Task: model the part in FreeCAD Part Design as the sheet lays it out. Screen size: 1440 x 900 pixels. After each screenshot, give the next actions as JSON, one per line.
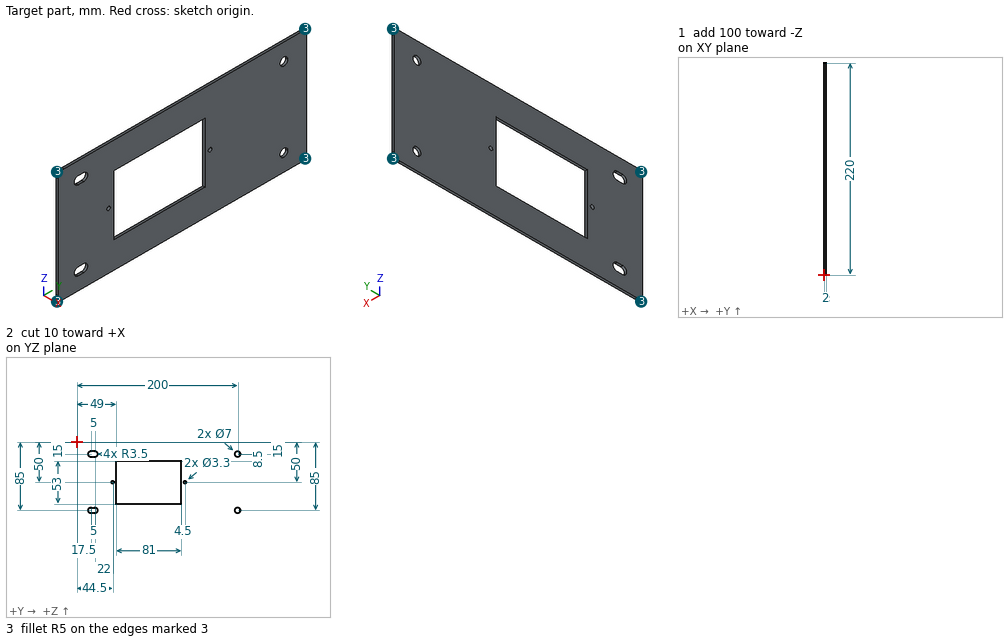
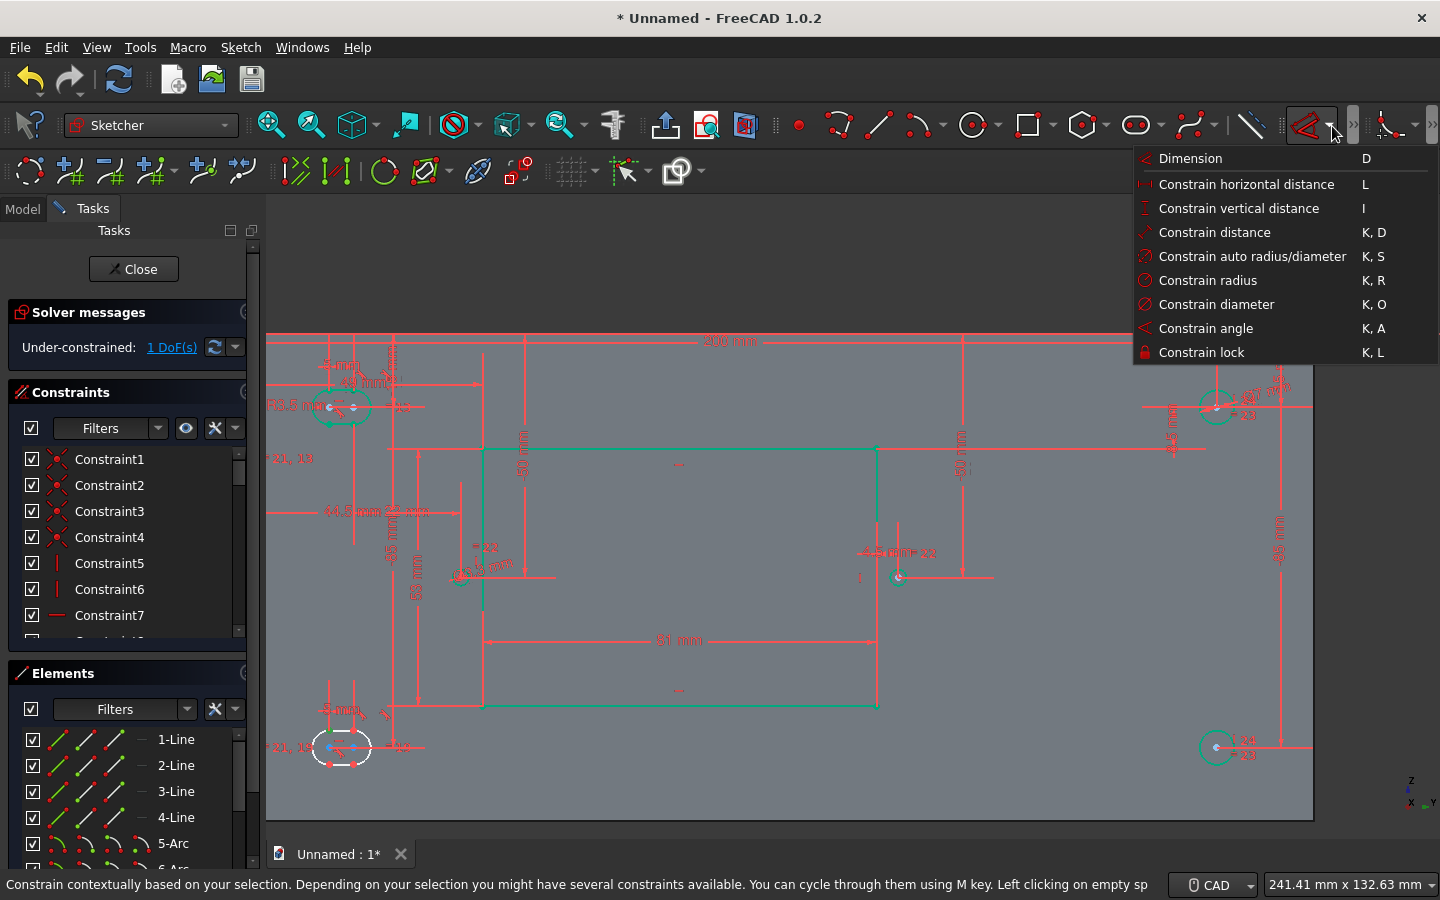
{"action": "left_click", "coordinate": [1286, 184]}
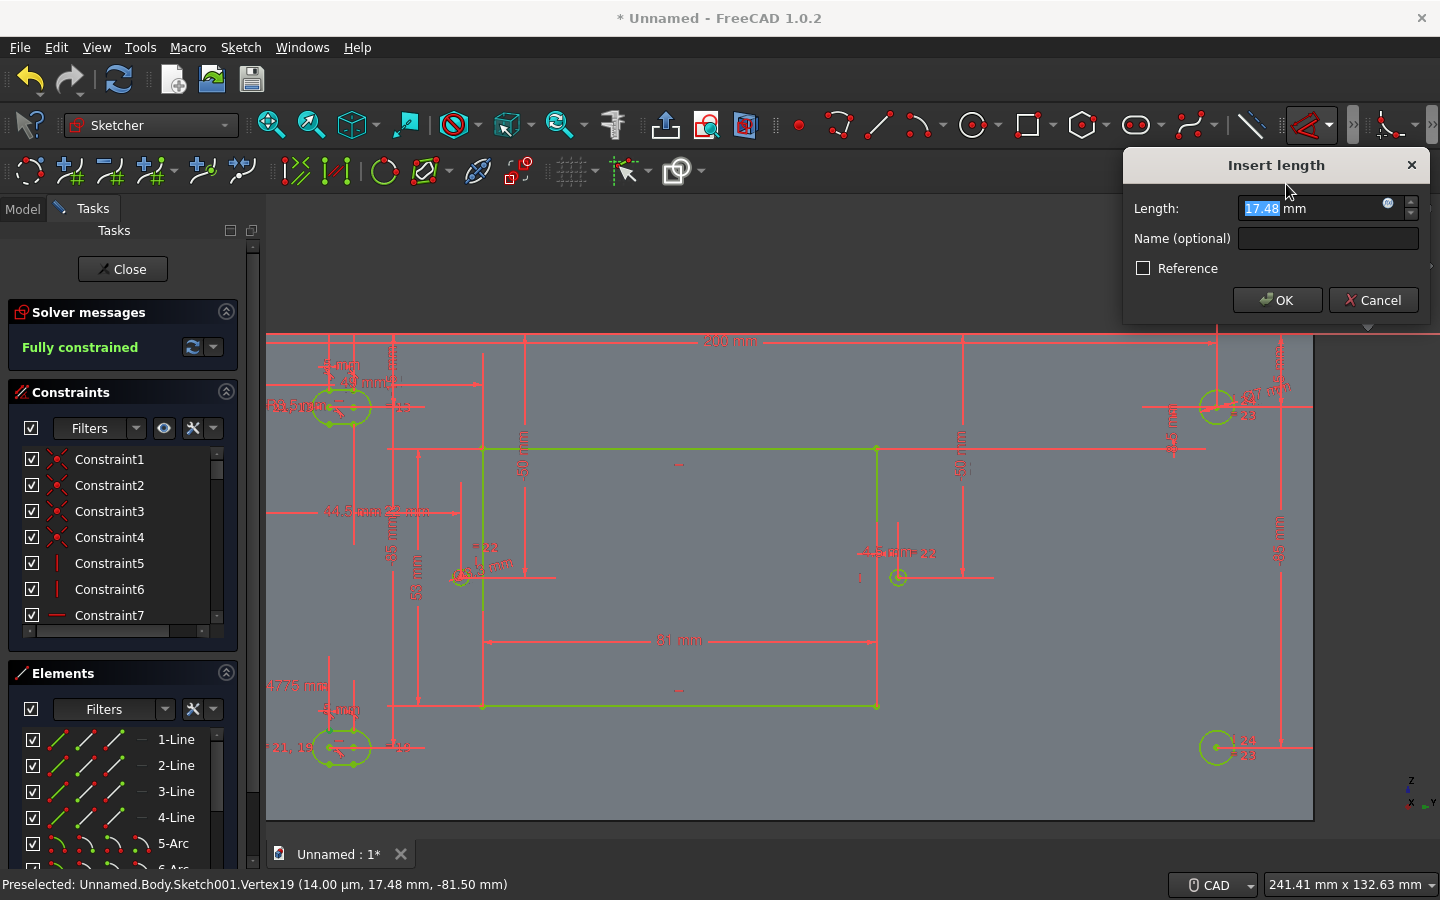
{"action": "type", "text": "17.5"}
{"action": "key", "text": "Return"}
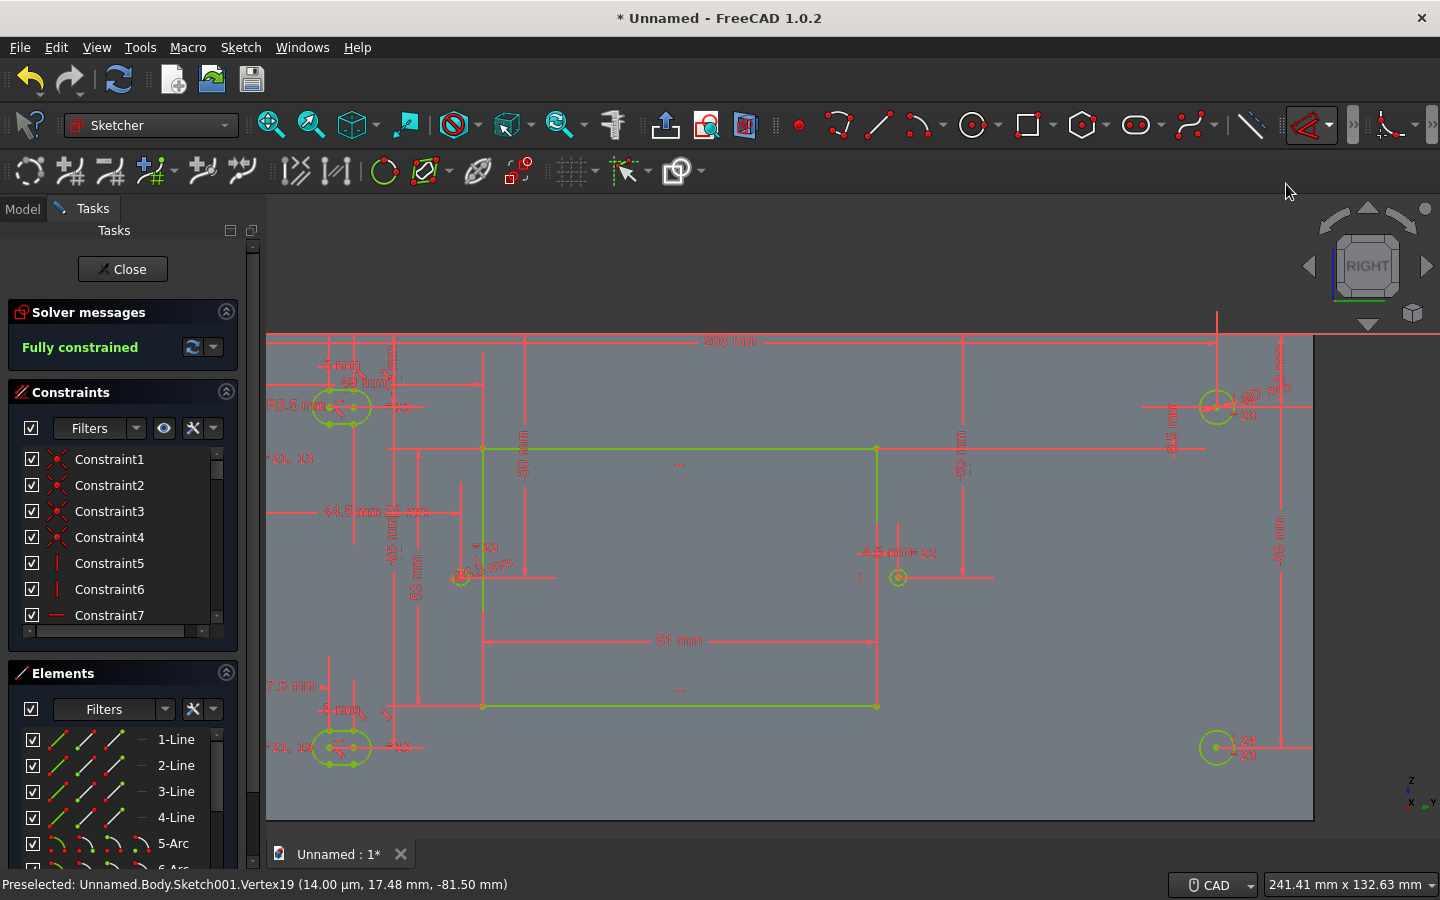
{"action": "left_click", "coordinate": [123, 269]}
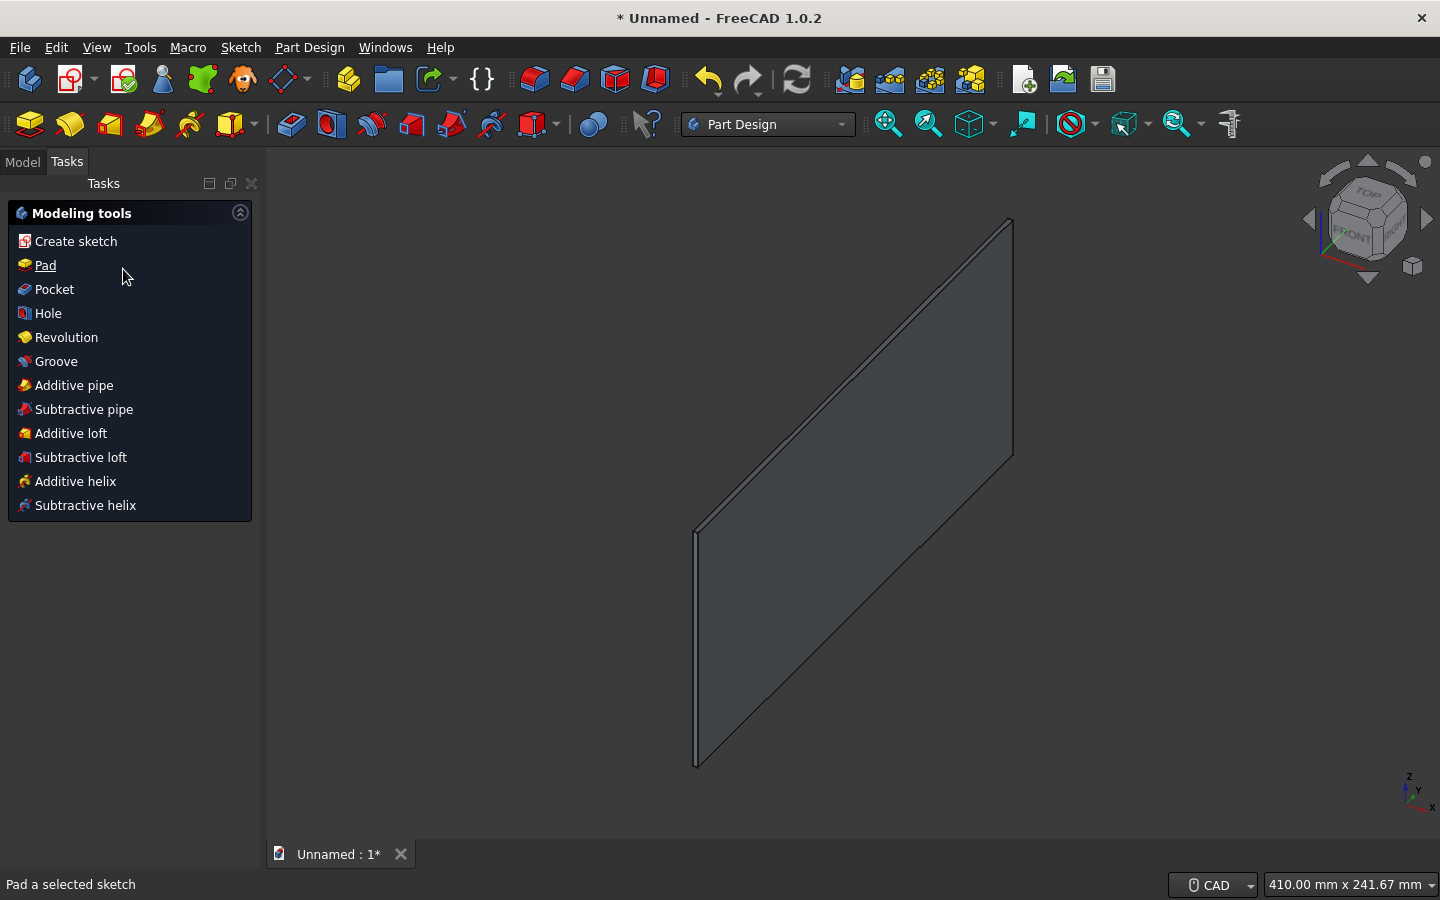
{"action": "left_click", "coordinate": [292, 124]}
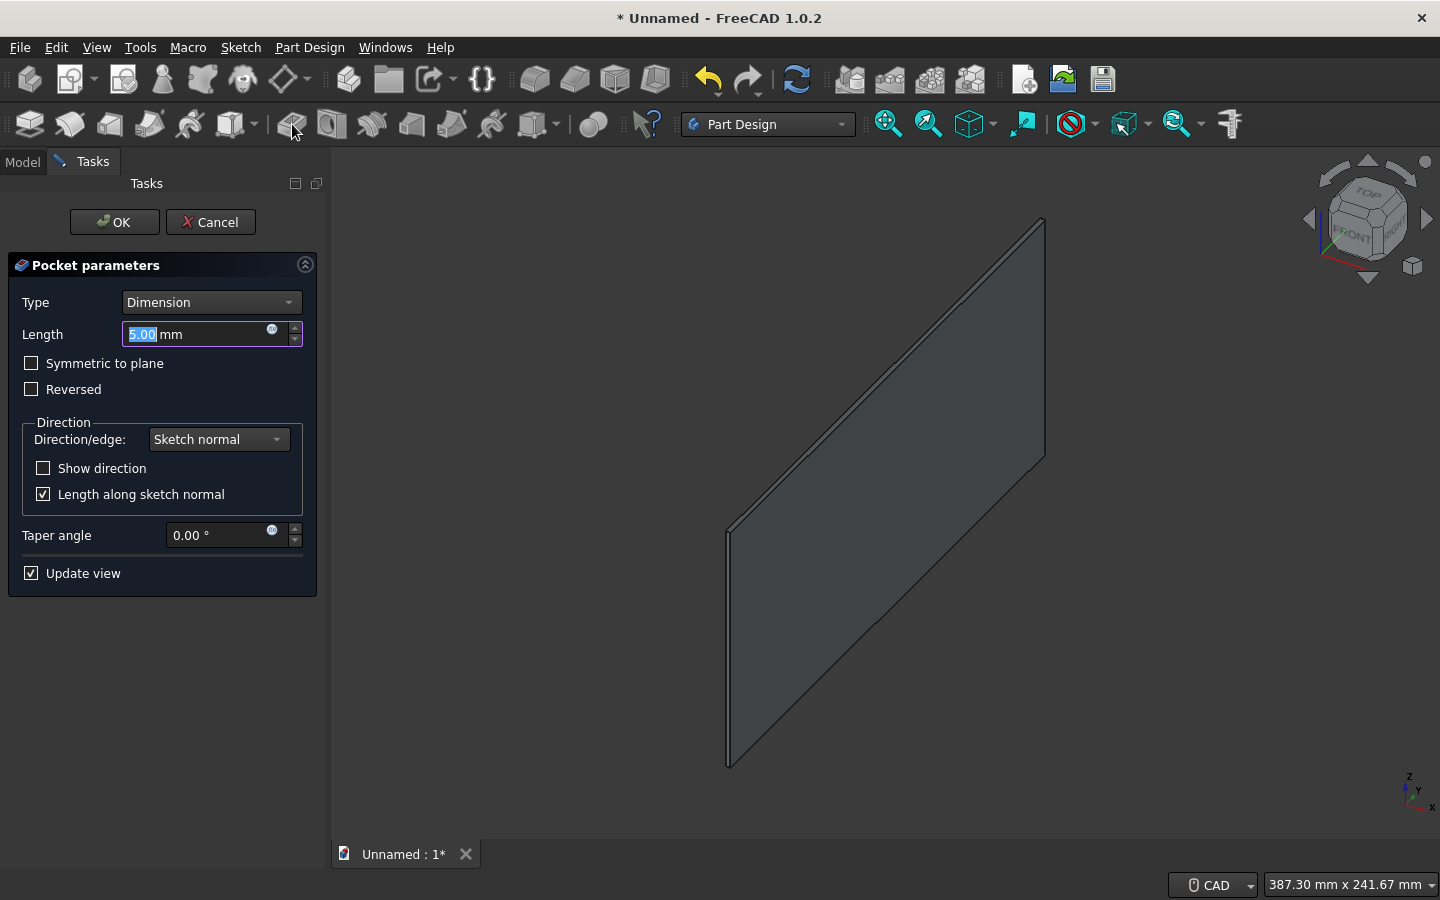
{"action": "type", "text": "10"}
{"action": "key", "text": "Tab"}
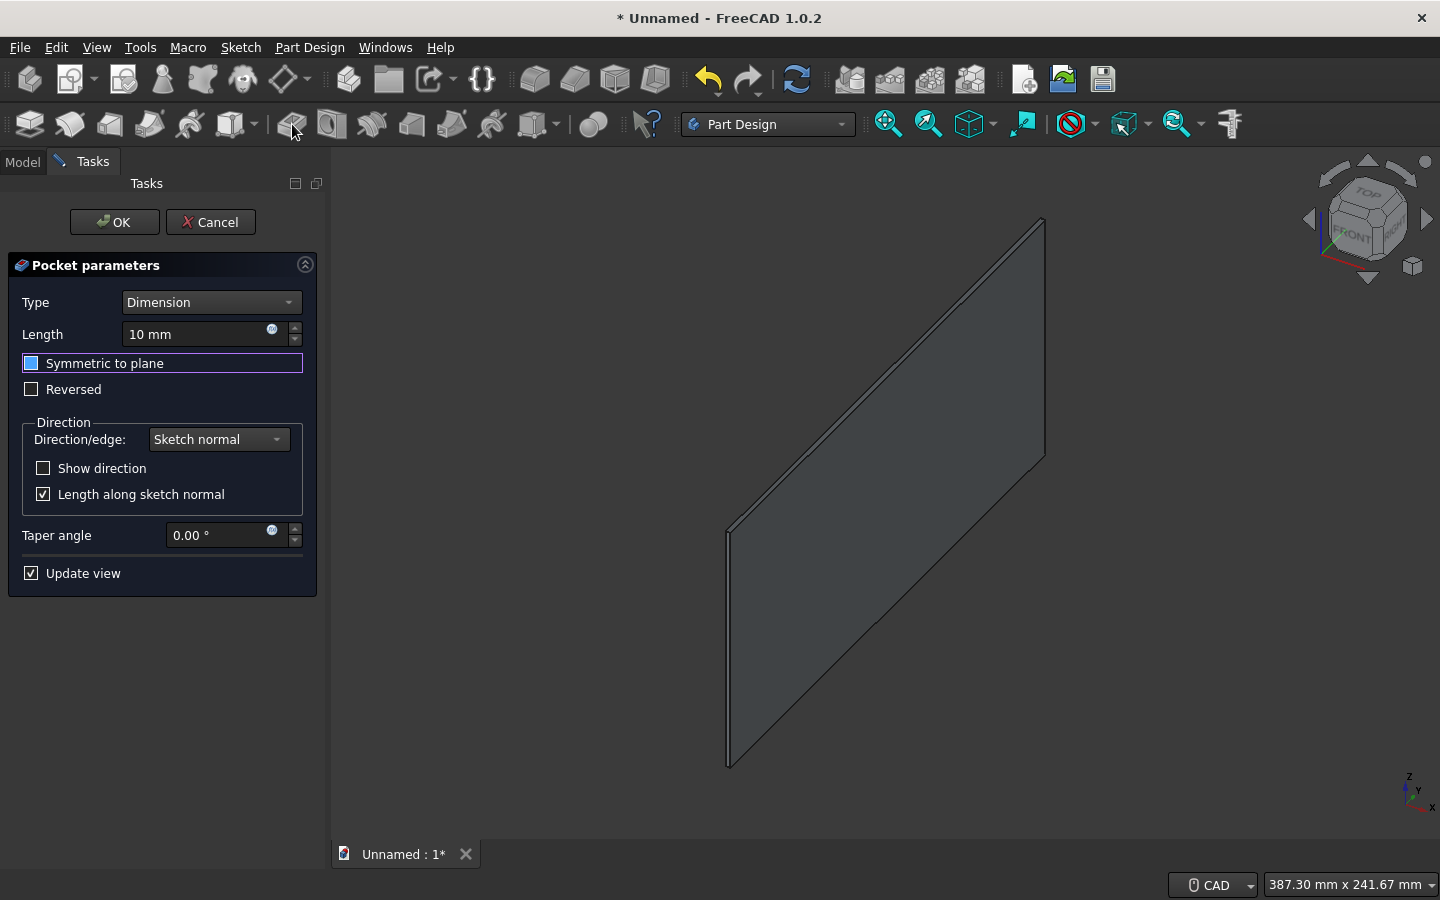
{"action": "left_click", "coordinate": [30, 389]}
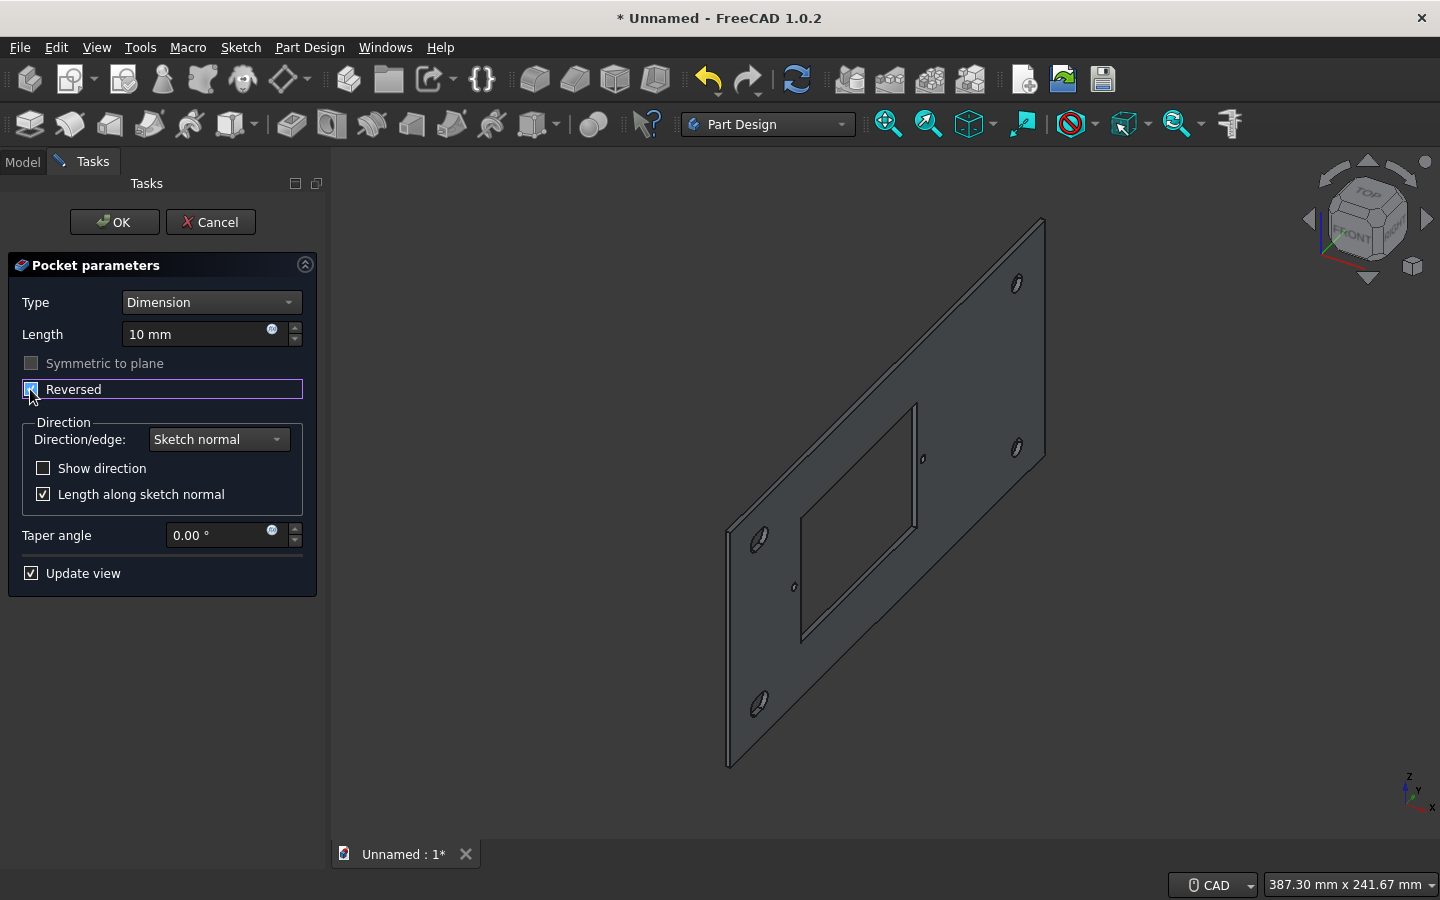
{"action": "left_click", "coordinate": [115, 222]}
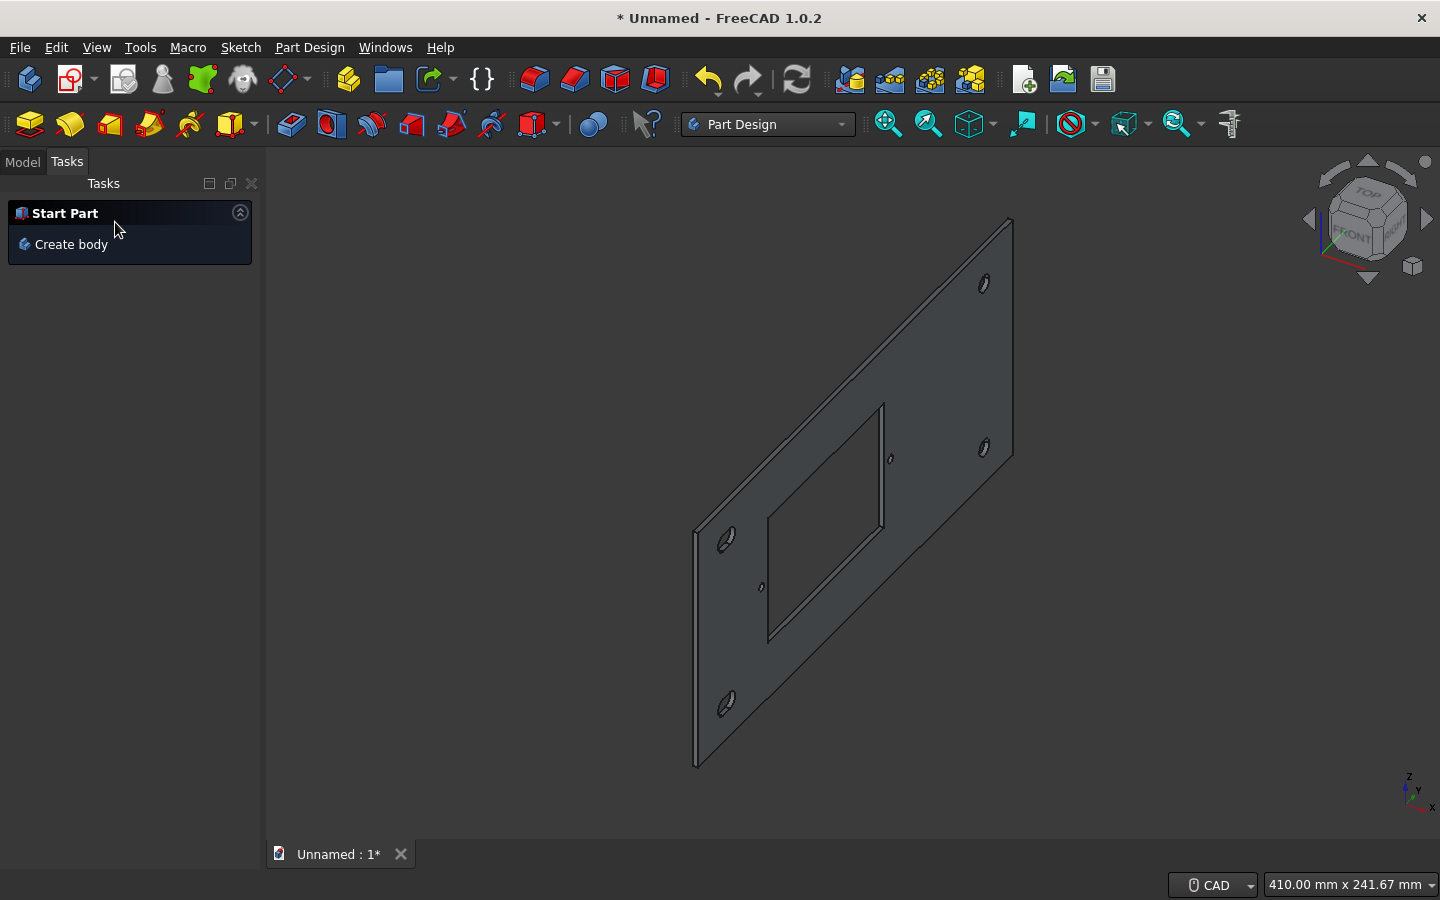
{"action": "scroll", "coordinate": [1010, 453], "scroll_direction": "up", "scroll_amount": 10}